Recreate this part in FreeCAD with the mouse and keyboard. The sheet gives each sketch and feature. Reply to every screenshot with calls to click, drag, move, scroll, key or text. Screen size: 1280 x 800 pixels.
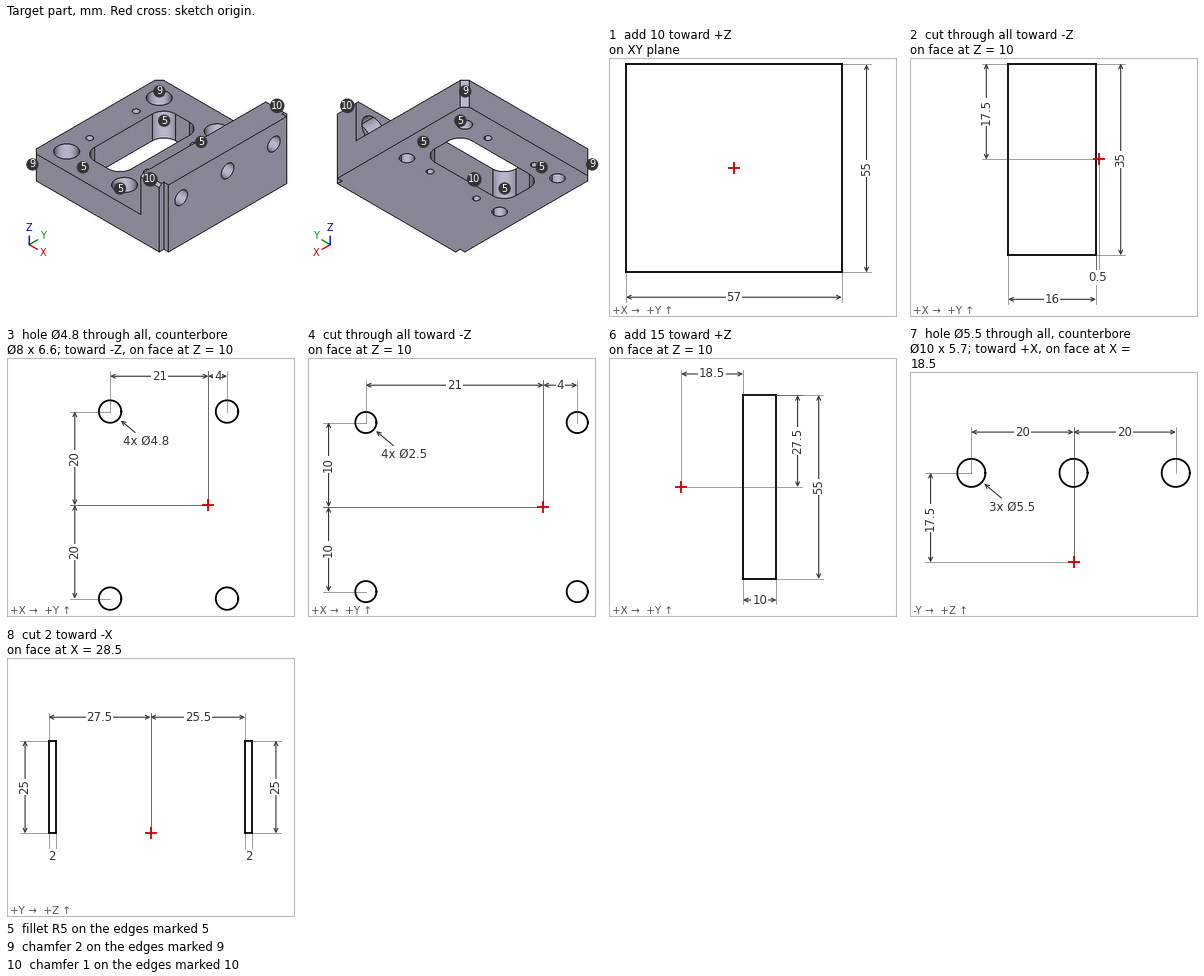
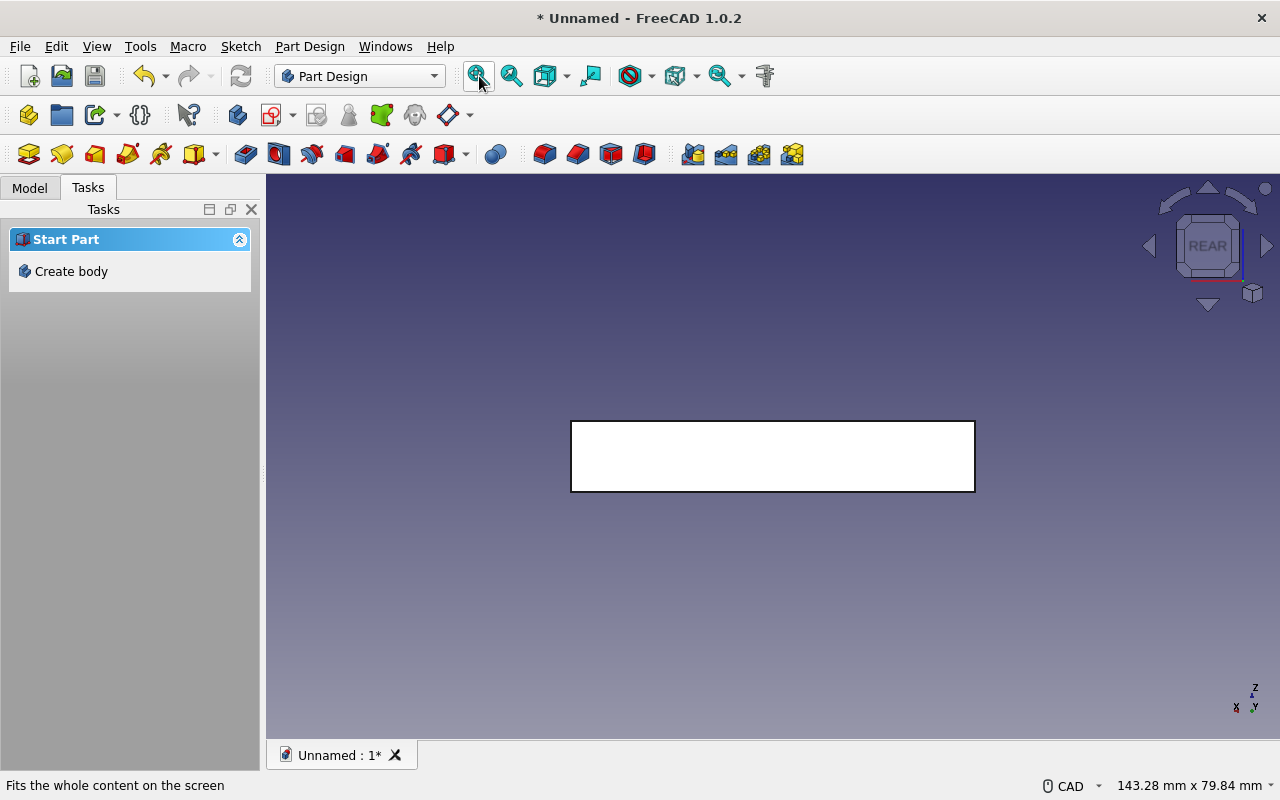
click(479, 76)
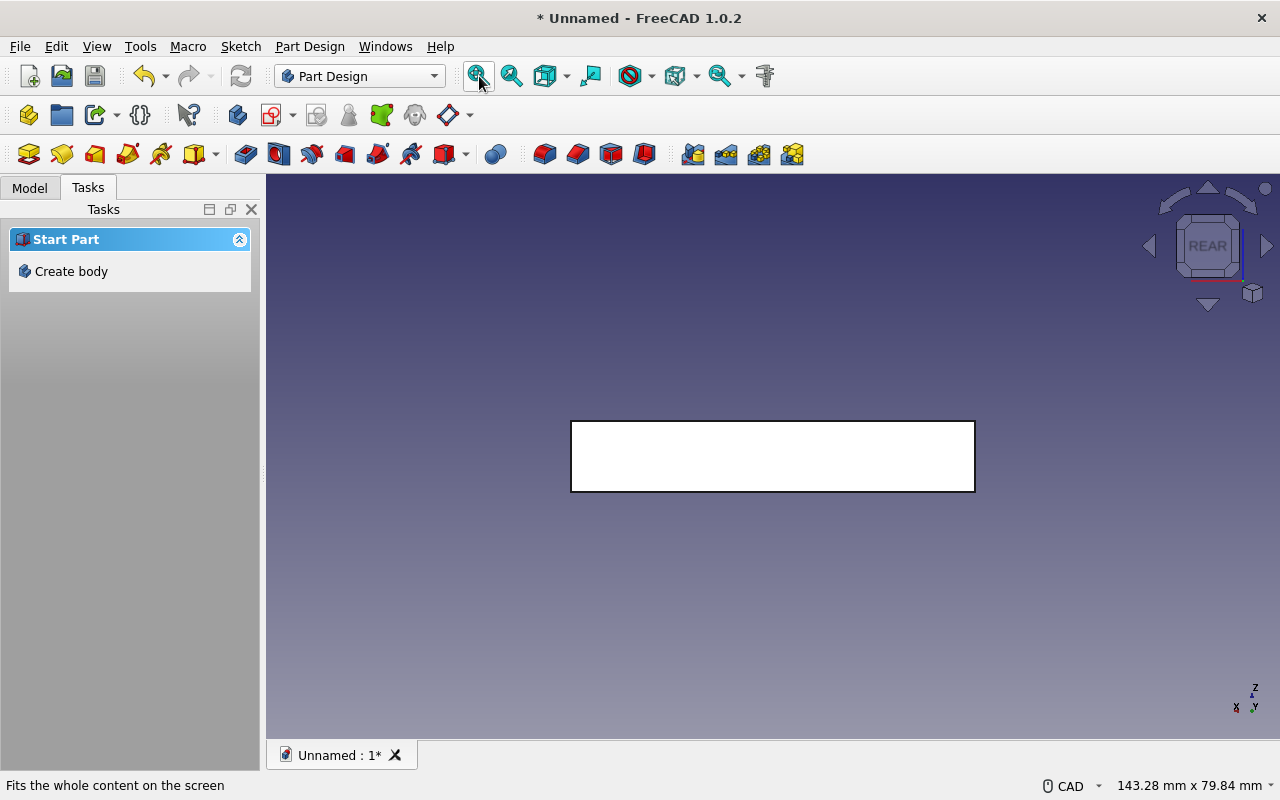
key(6)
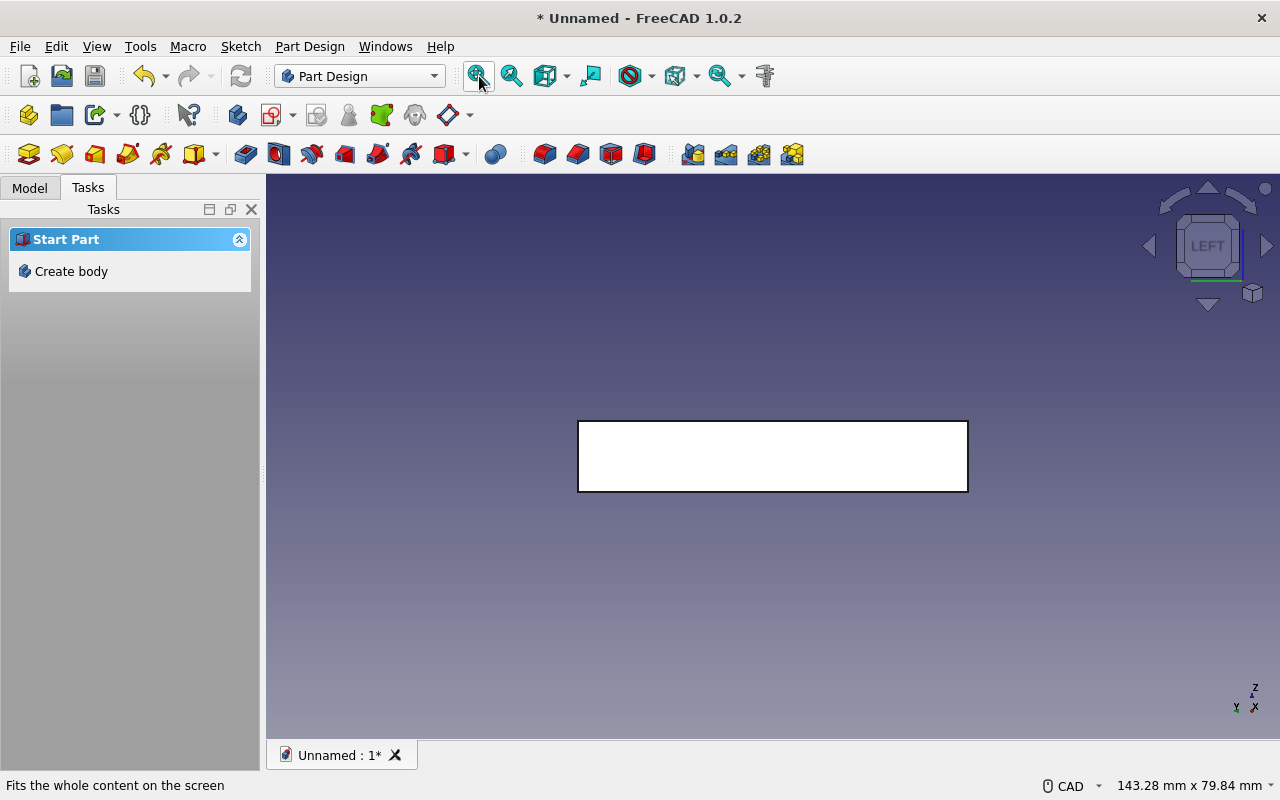
key(v)
key(f)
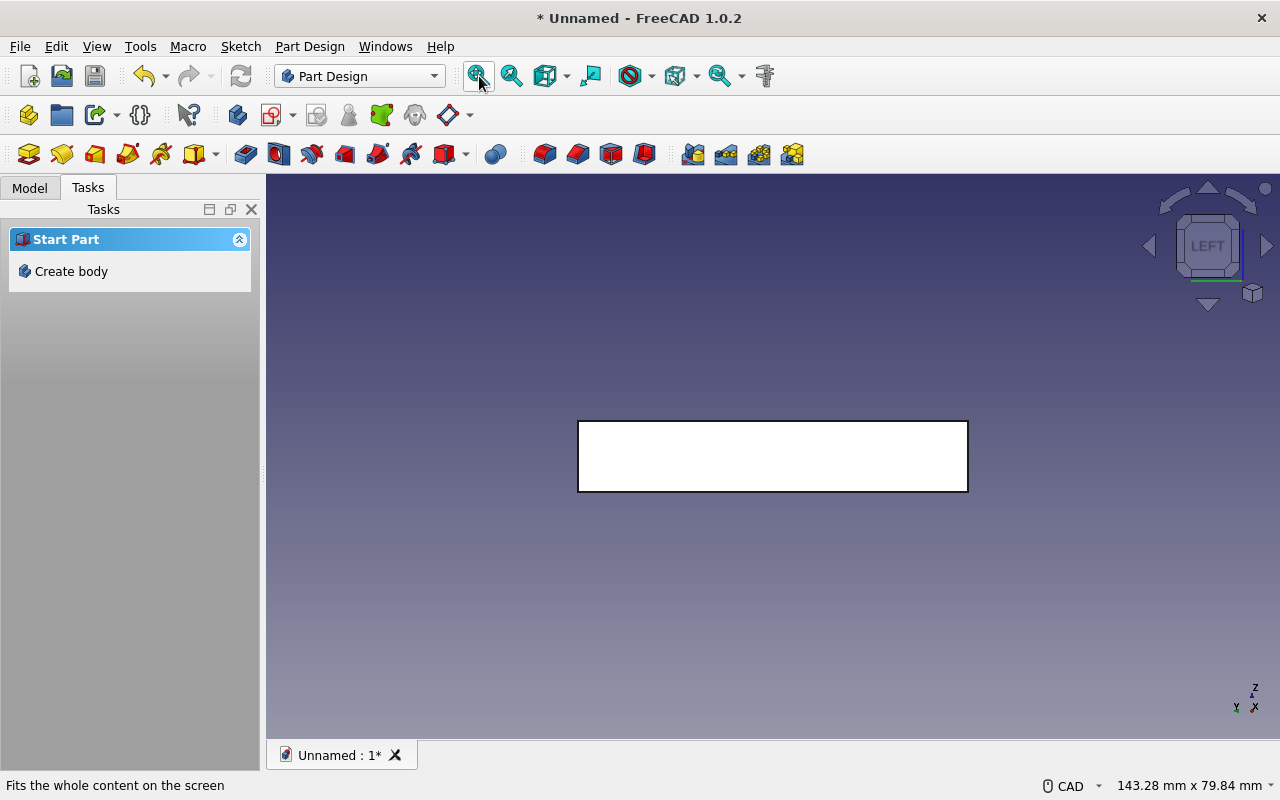
key(v)
key(3)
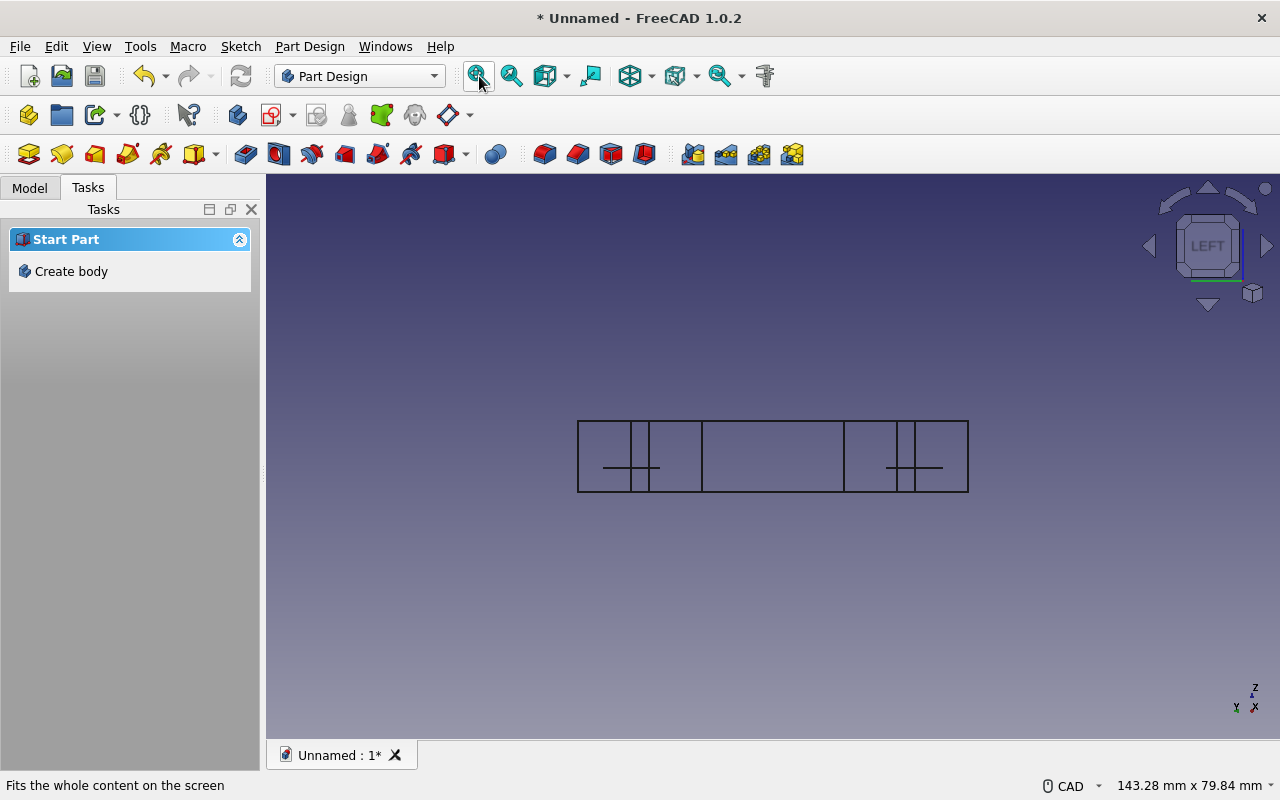
key(0)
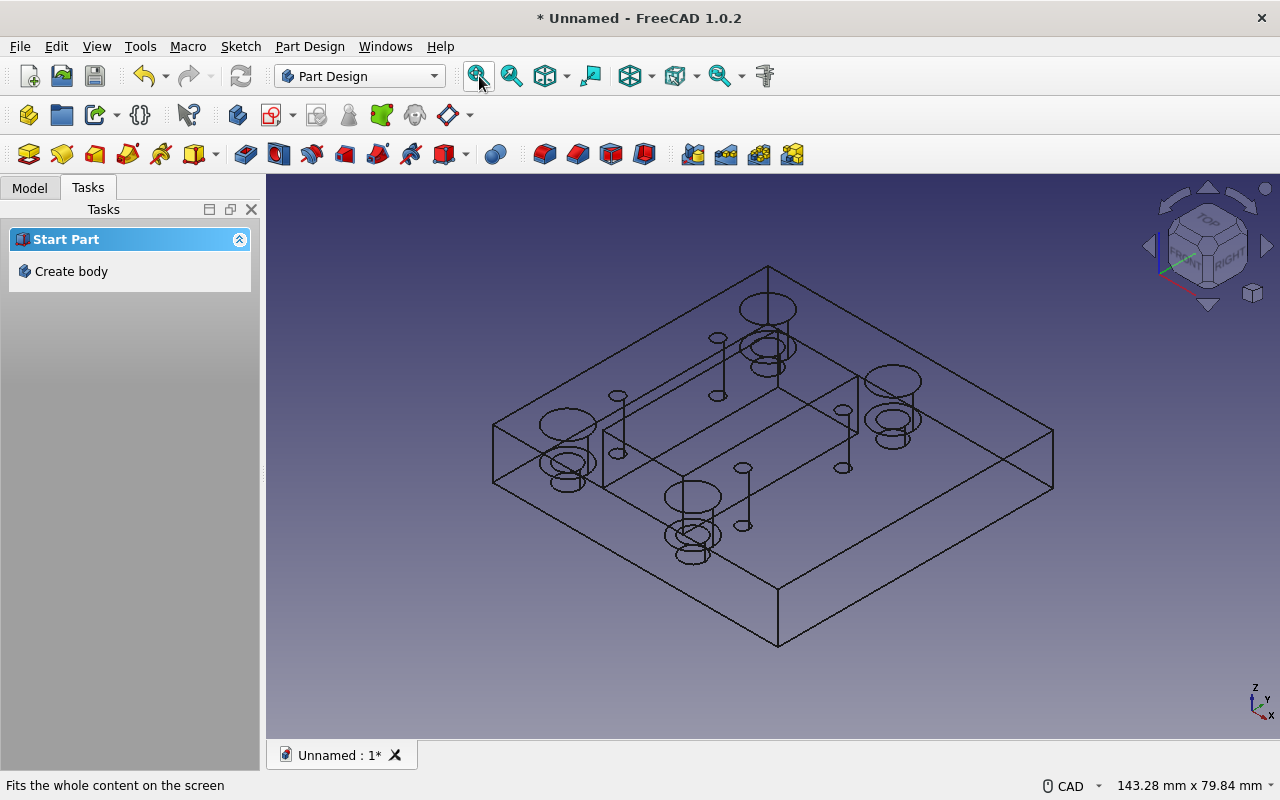
click(603, 458)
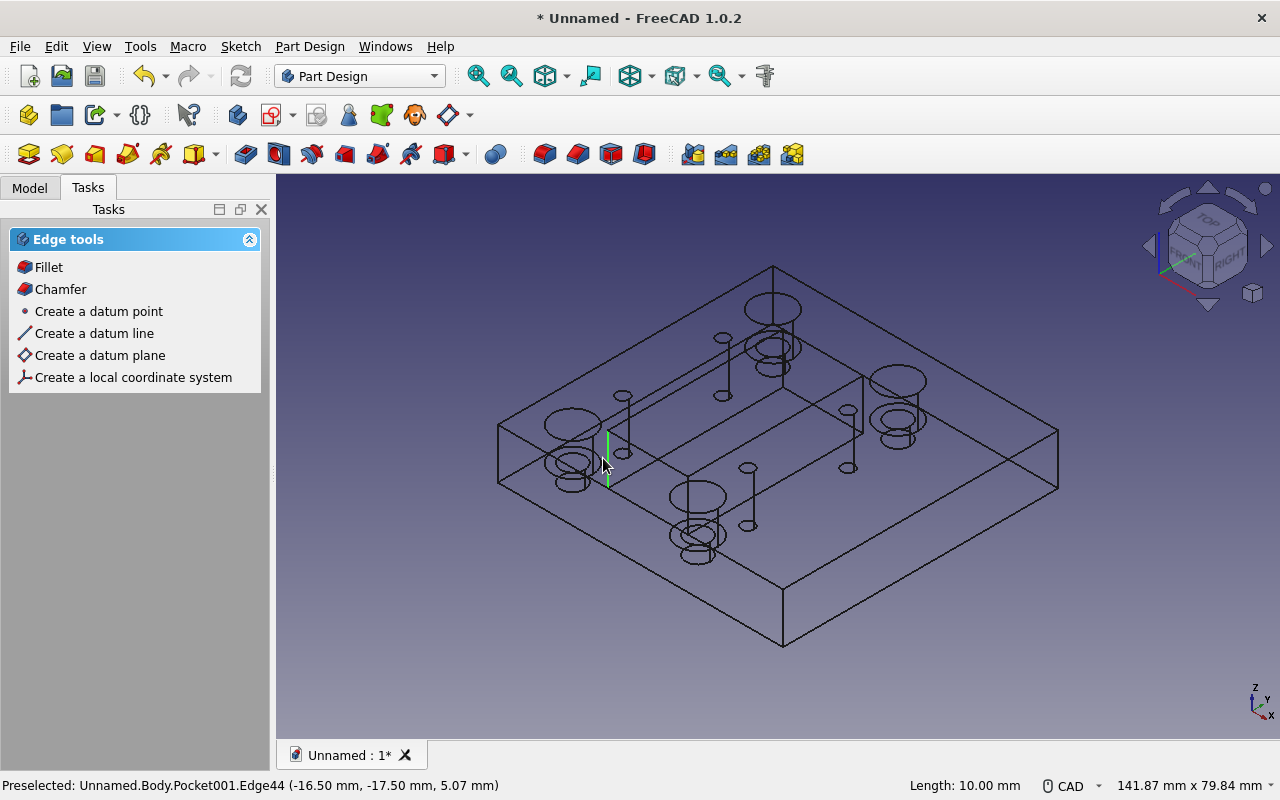
click(783, 357, ctrl)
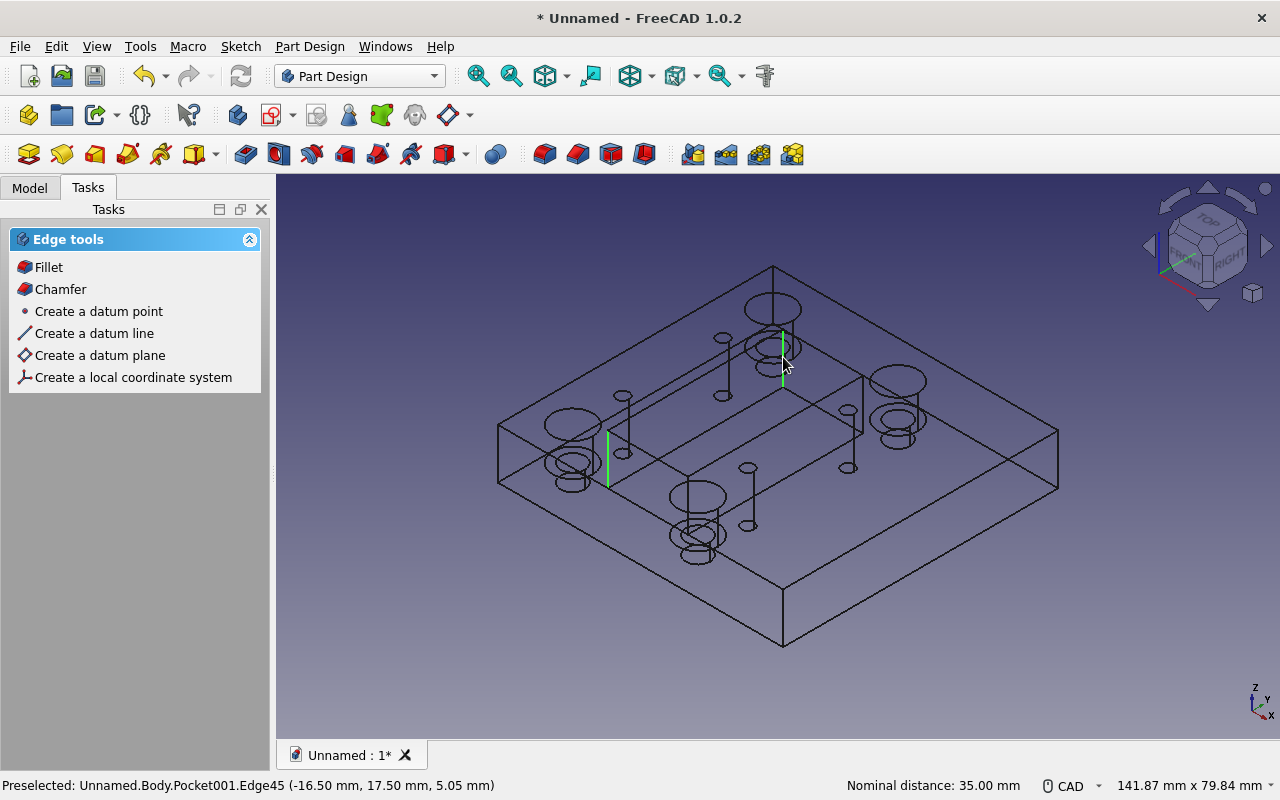
click(863, 403, ctrl)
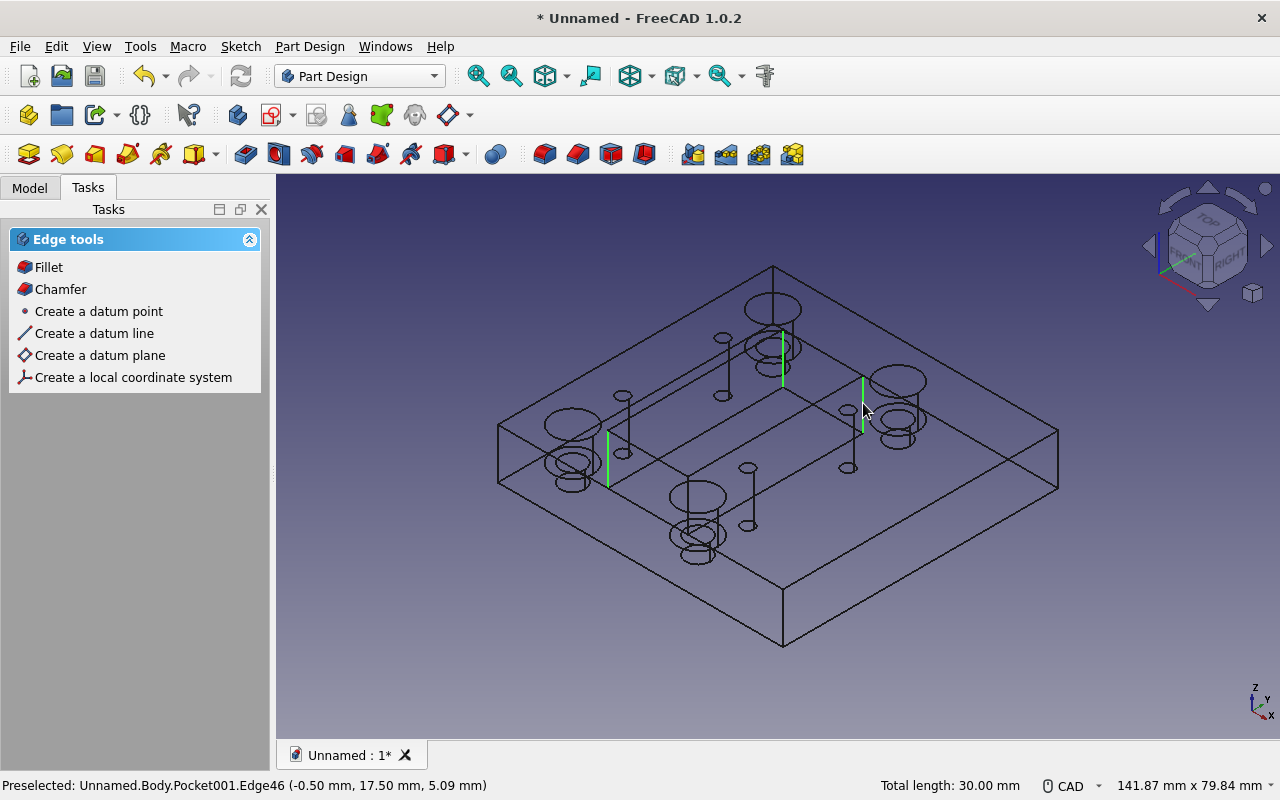
click(688, 499, ctrl)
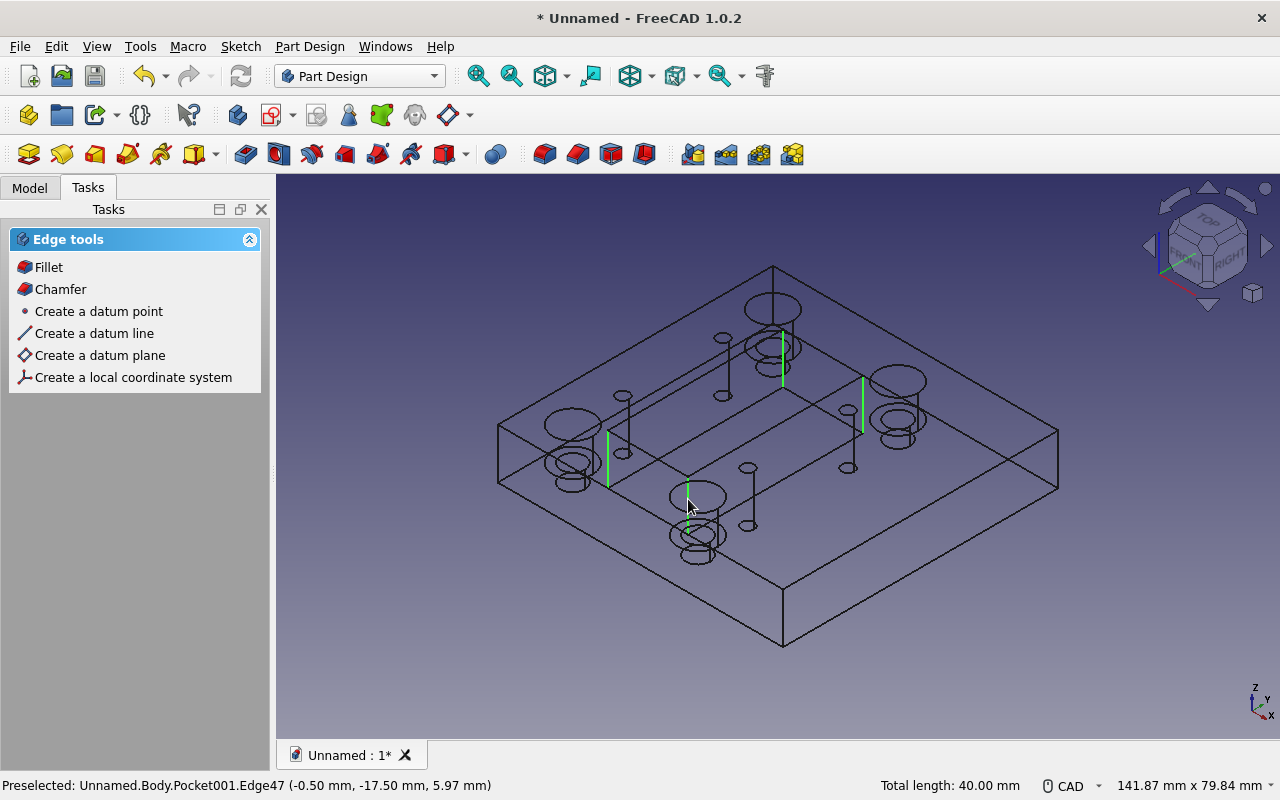
key(v)
key(1)